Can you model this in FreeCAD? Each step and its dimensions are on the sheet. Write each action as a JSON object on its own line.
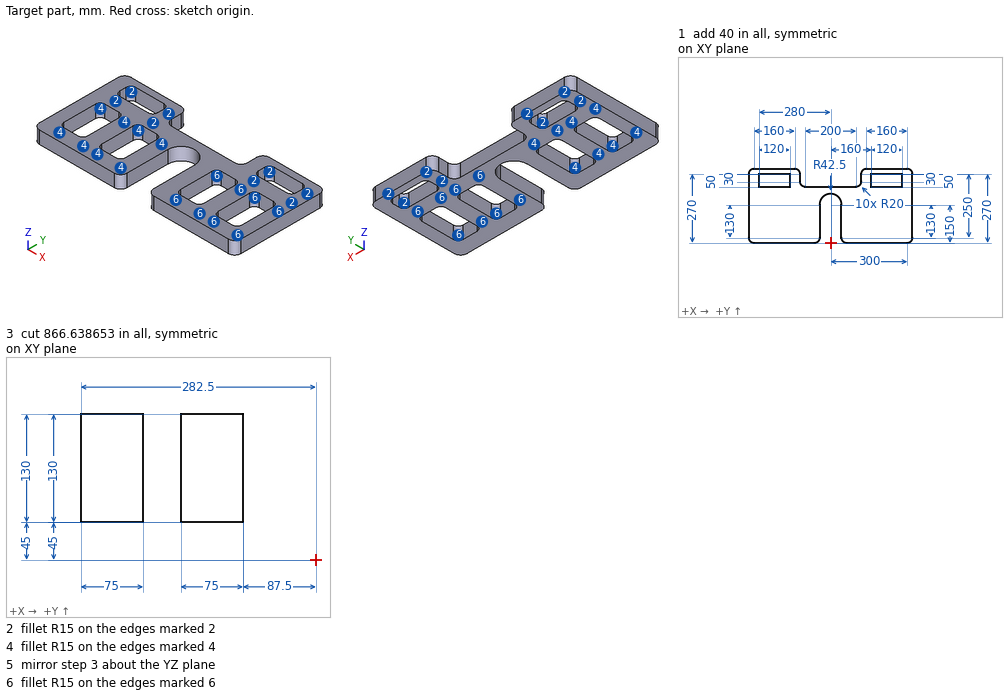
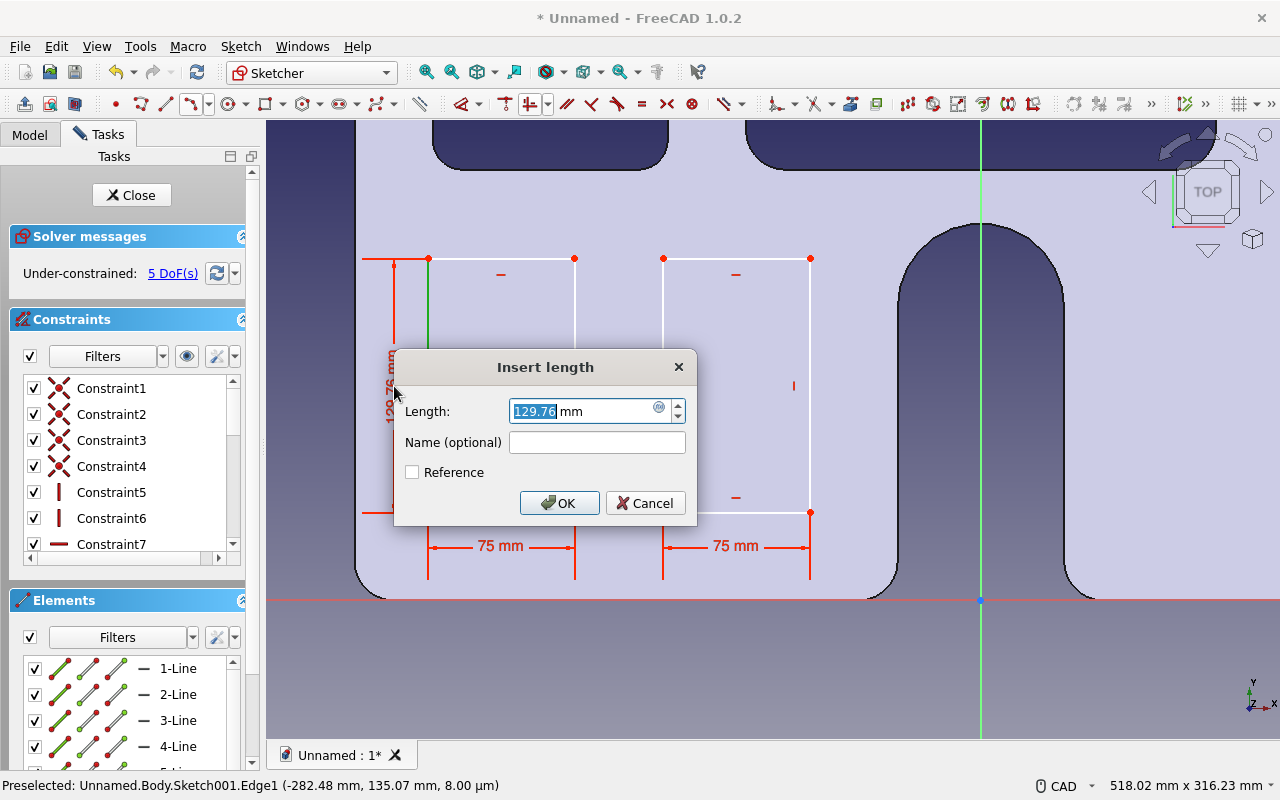
{"action": "type", "text": "130"}
{"action": "key", "text": "Return"}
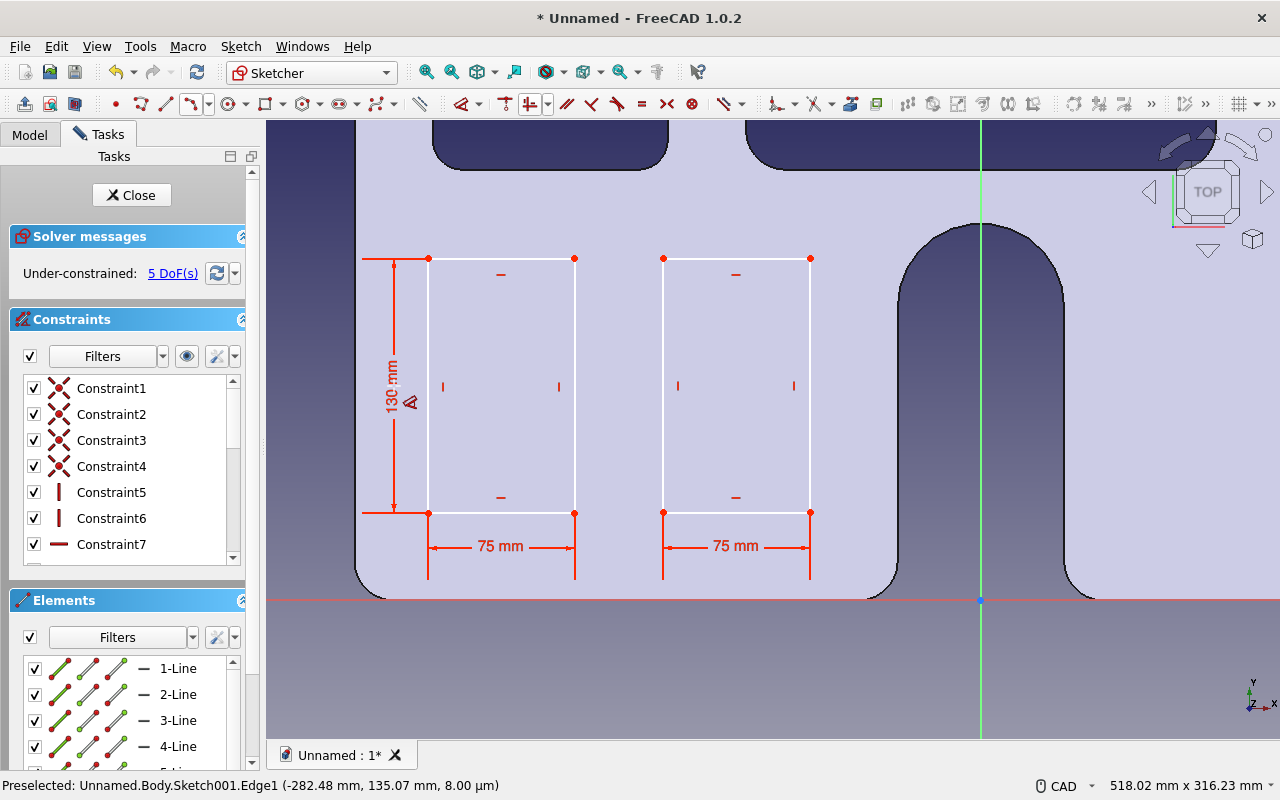
{"action": "left_click", "coordinate": [663, 335]}
{"action": "left_click", "coordinate": [629, 386]}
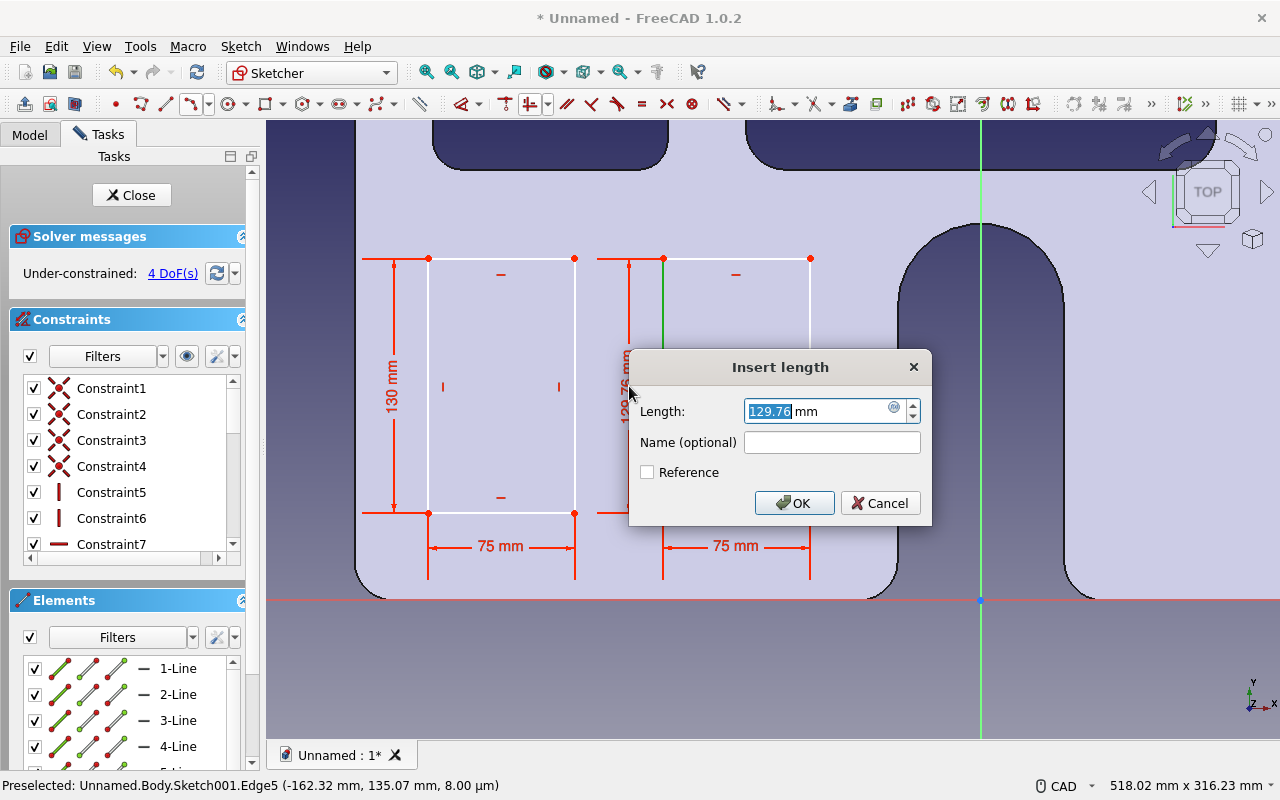
{"action": "type", "text": "130"}
{"action": "key", "text": "Return"}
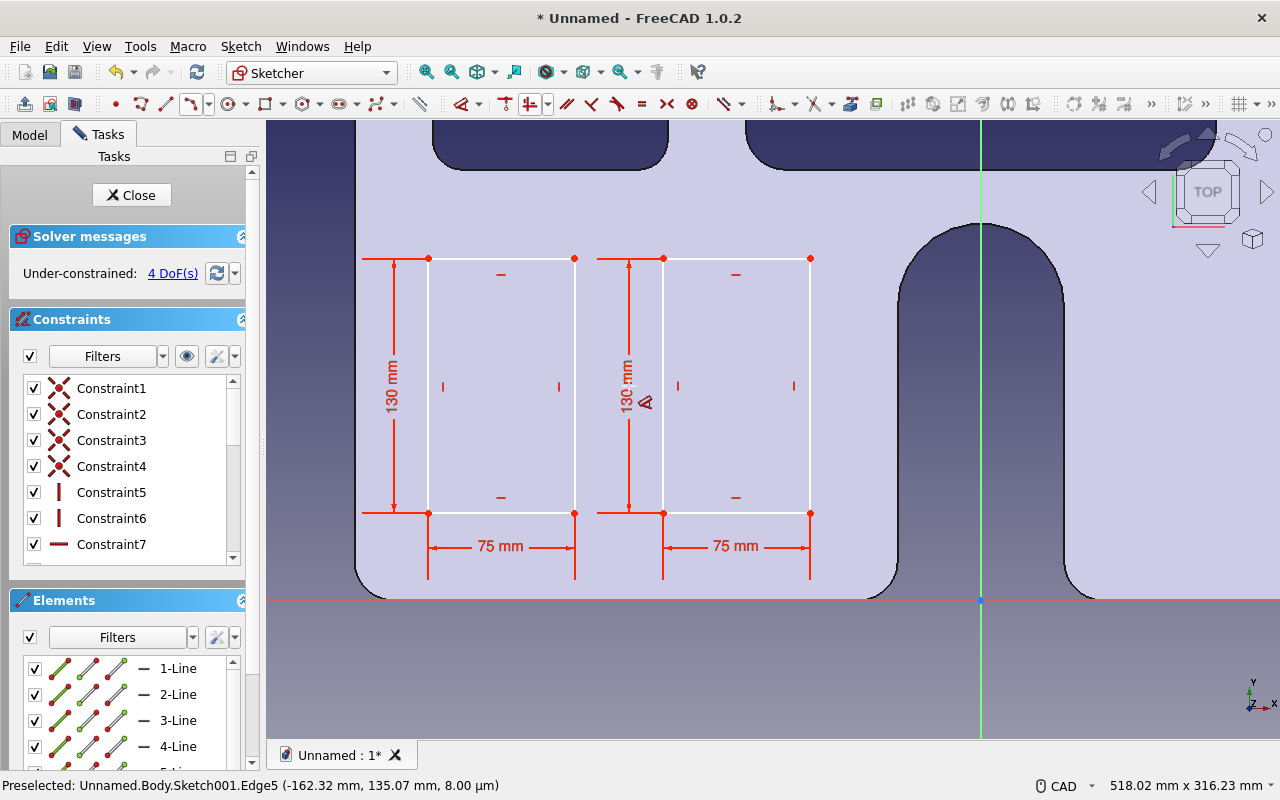
{"action": "left_click", "coordinate": [428, 513]}
{"action": "left_click", "coordinate": [1015, 557]}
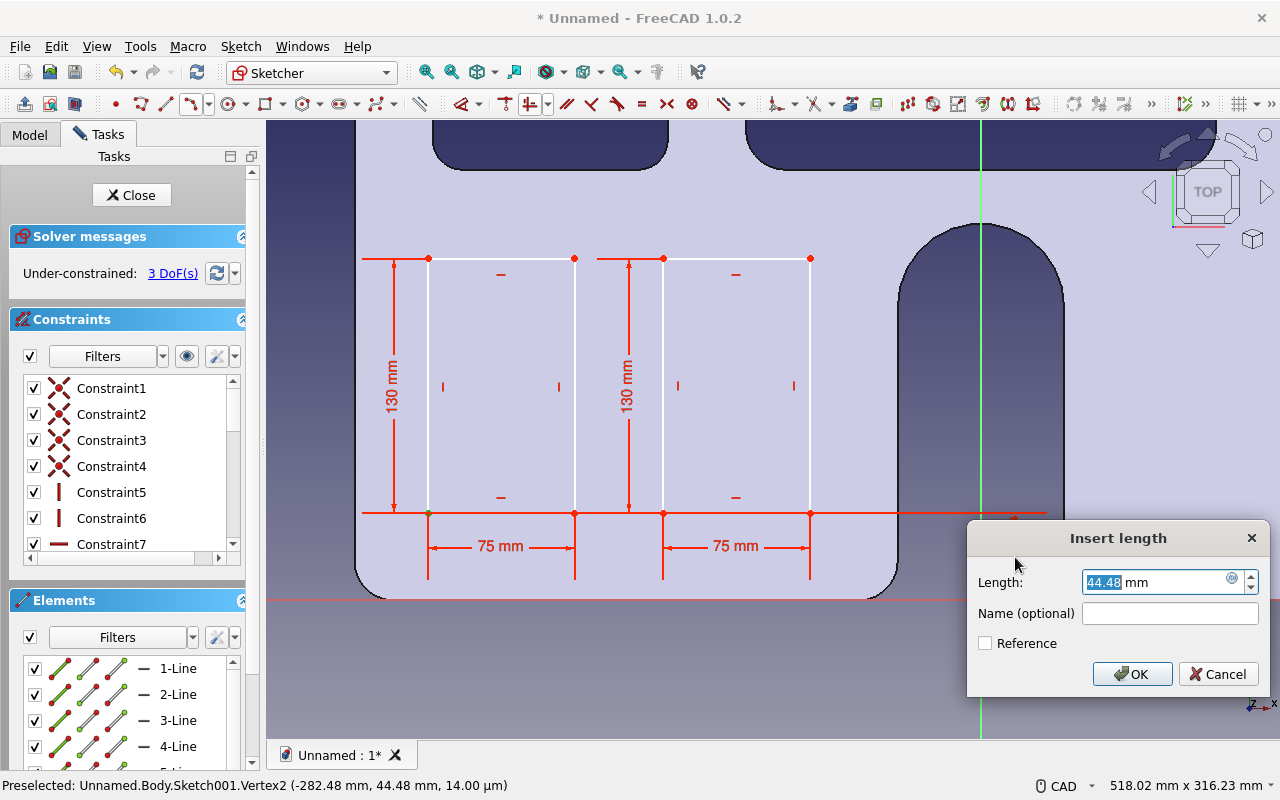
{"action": "type", "text": "45"}
{"action": "key", "text": "Return"}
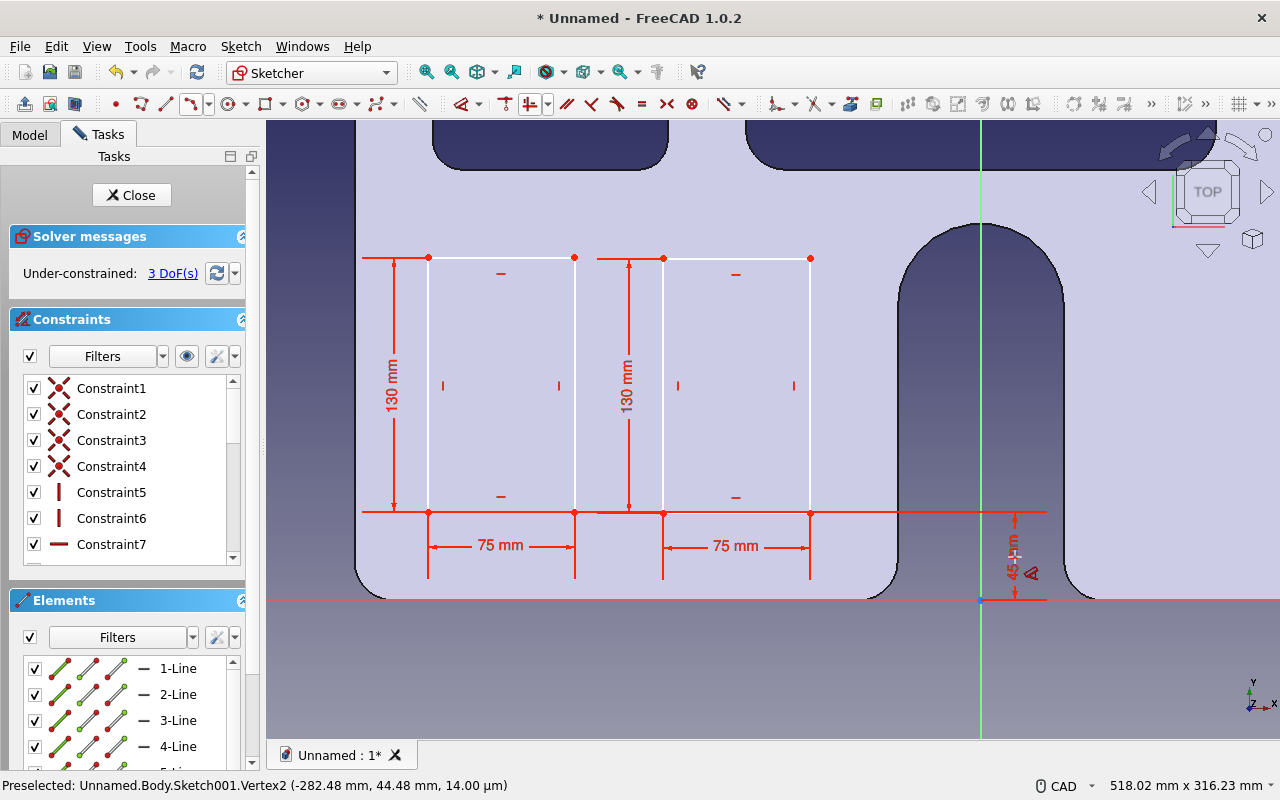
{"action": "left_click", "coordinate": [663, 513]}
{"action": "left_click", "coordinate": [1015, 537]}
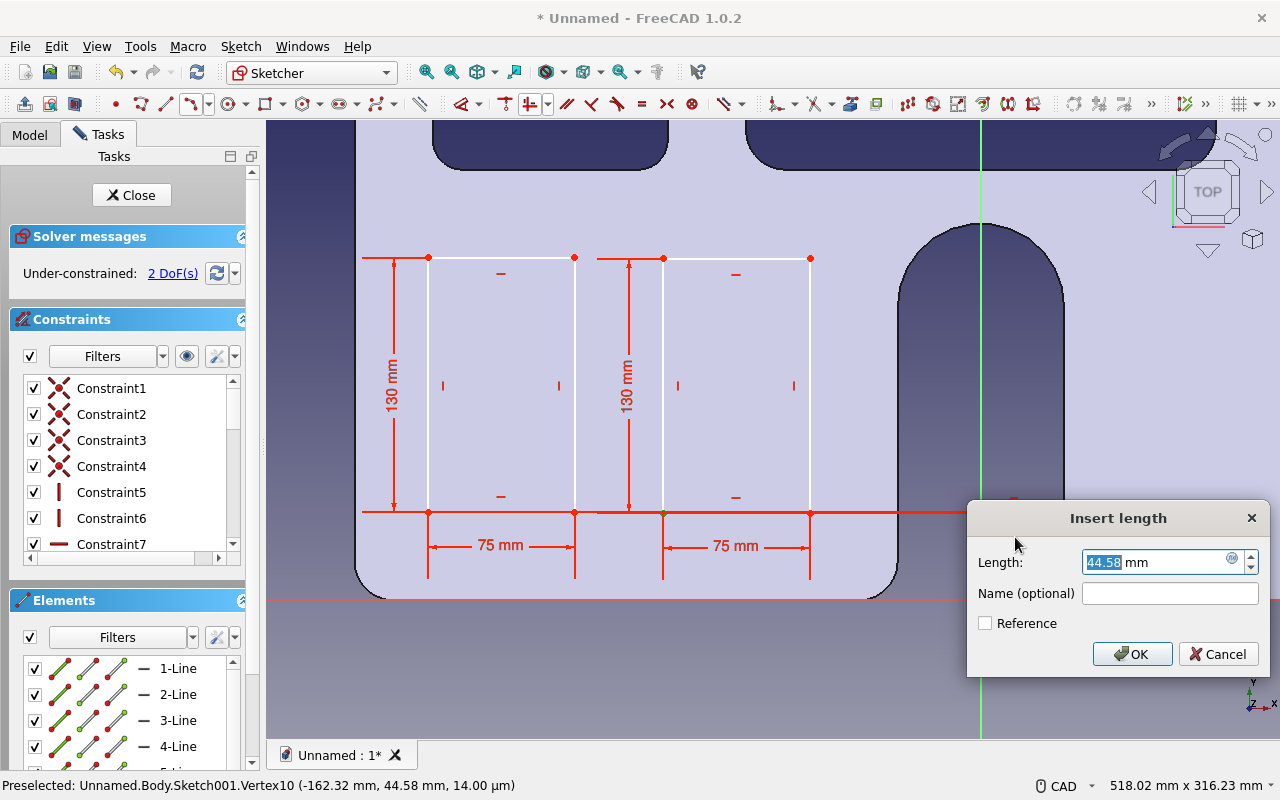
{"action": "type", "text": "45"}
{"action": "key", "text": "Return"}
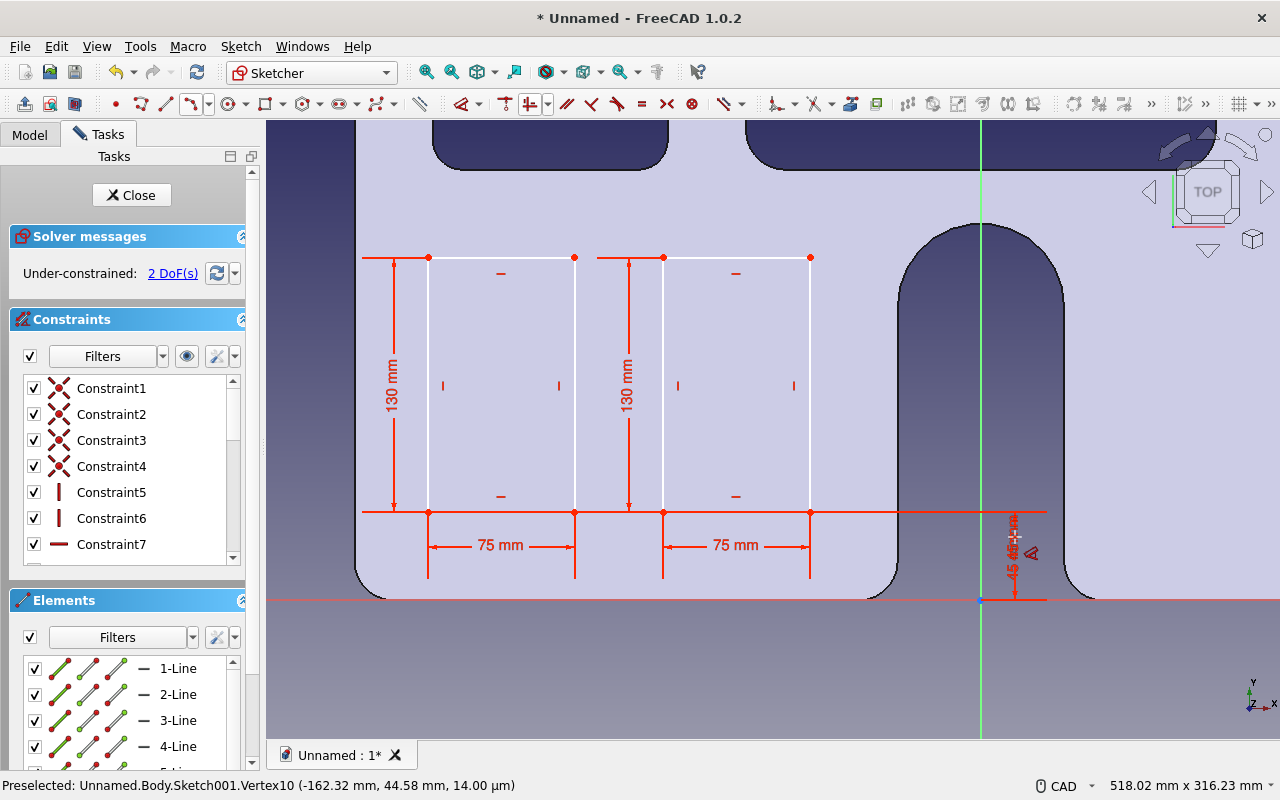
{"action": "left_click", "coordinate": [810, 512]}
{"action": "left_click", "coordinate": [895, 634]}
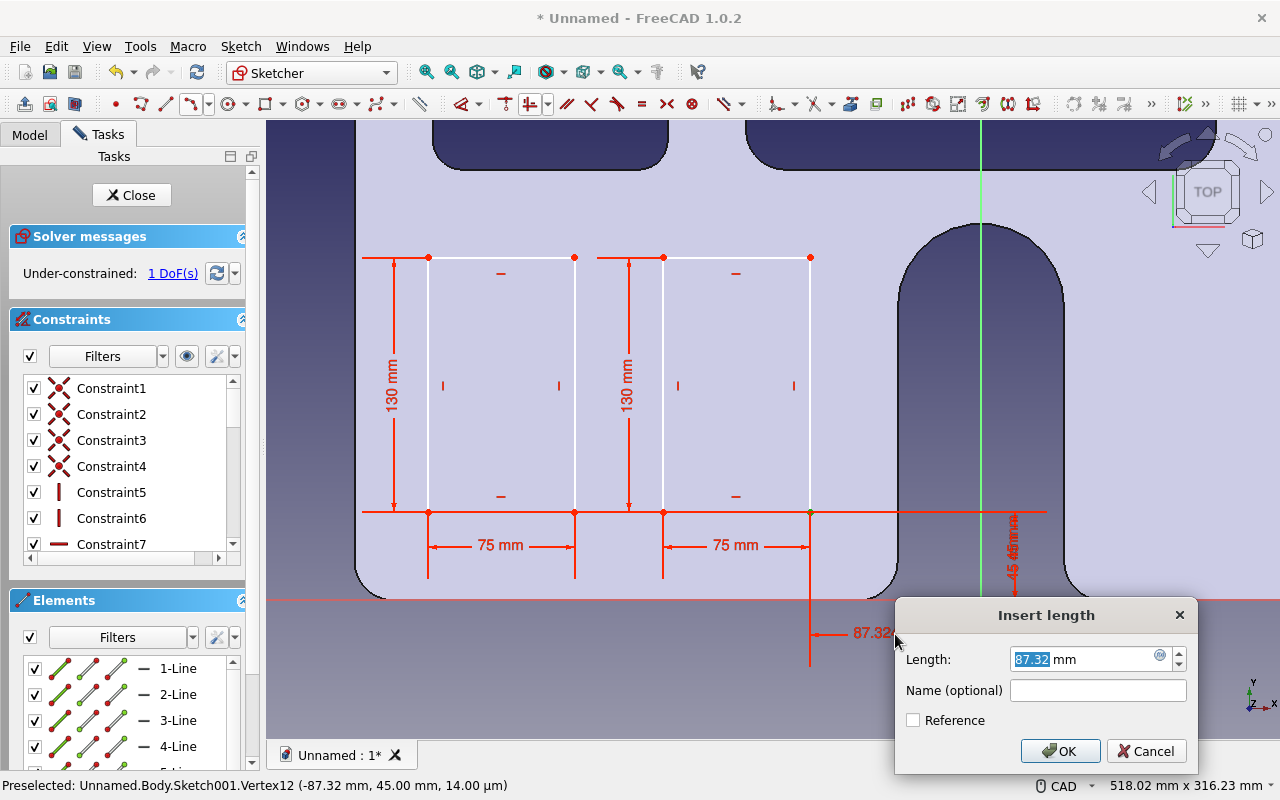
{"action": "type", "text": "87.5"}
{"action": "key", "text": "Return"}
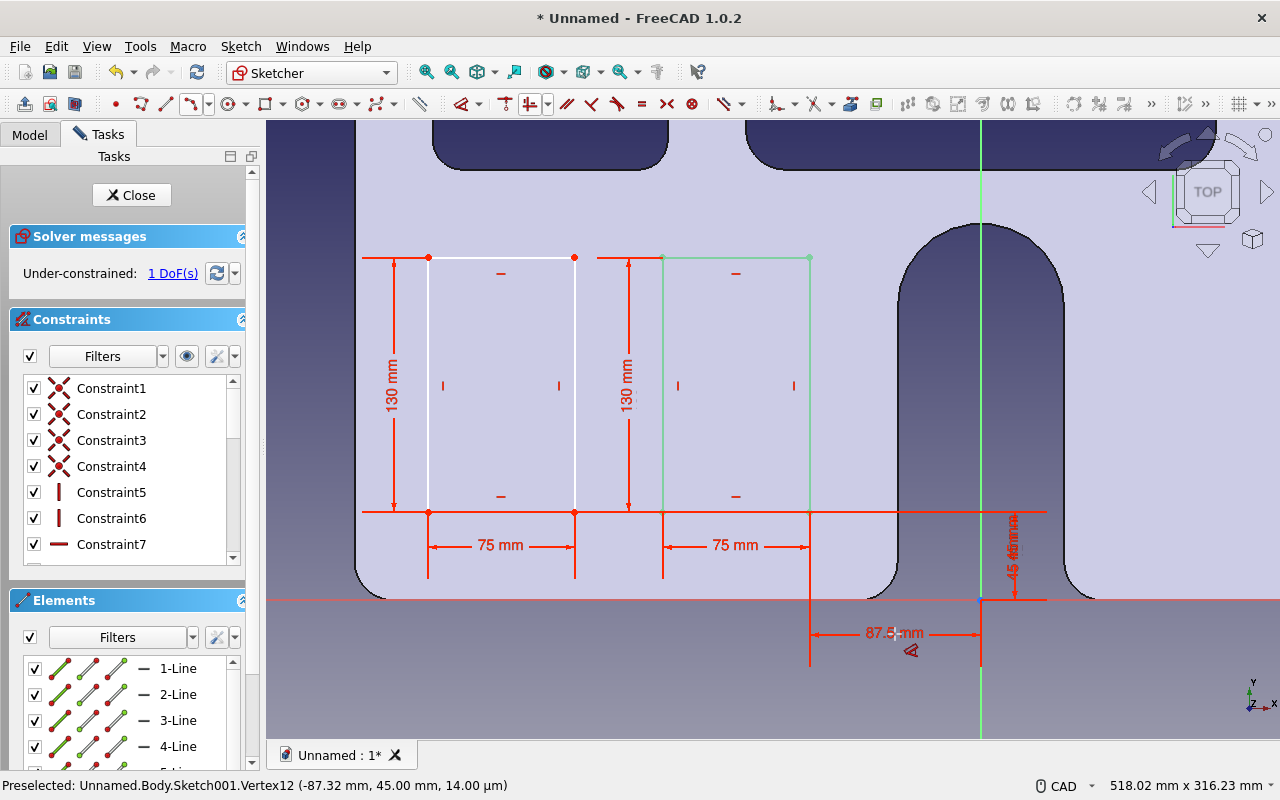
{"action": "left_click", "coordinate": [428, 258]}
{"action": "left_click", "coordinate": [704, 634]}